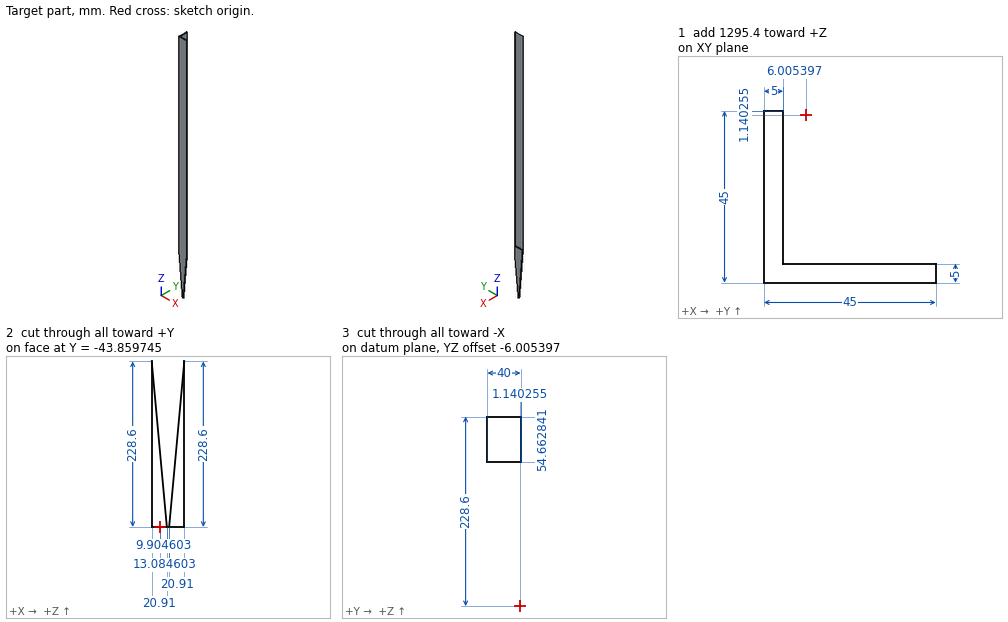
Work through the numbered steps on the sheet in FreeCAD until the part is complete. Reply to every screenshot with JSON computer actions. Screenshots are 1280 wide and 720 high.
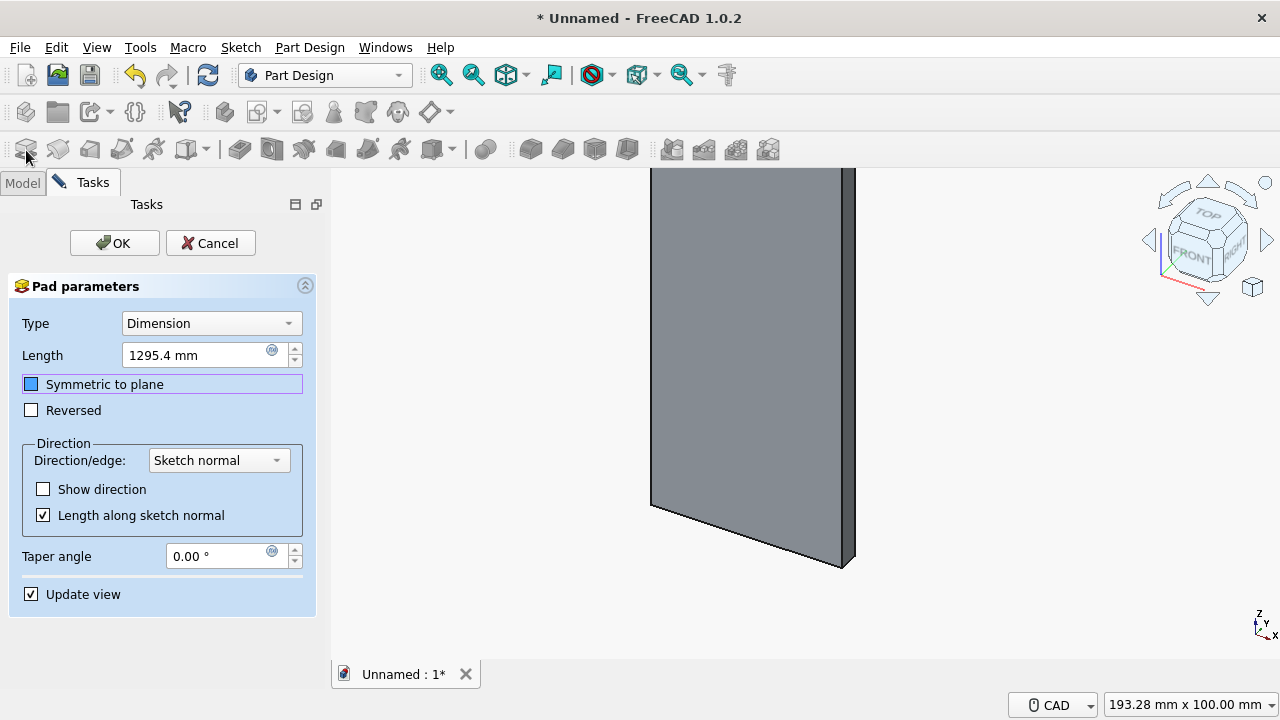
{"action": "left_click", "coordinate": [115, 243]}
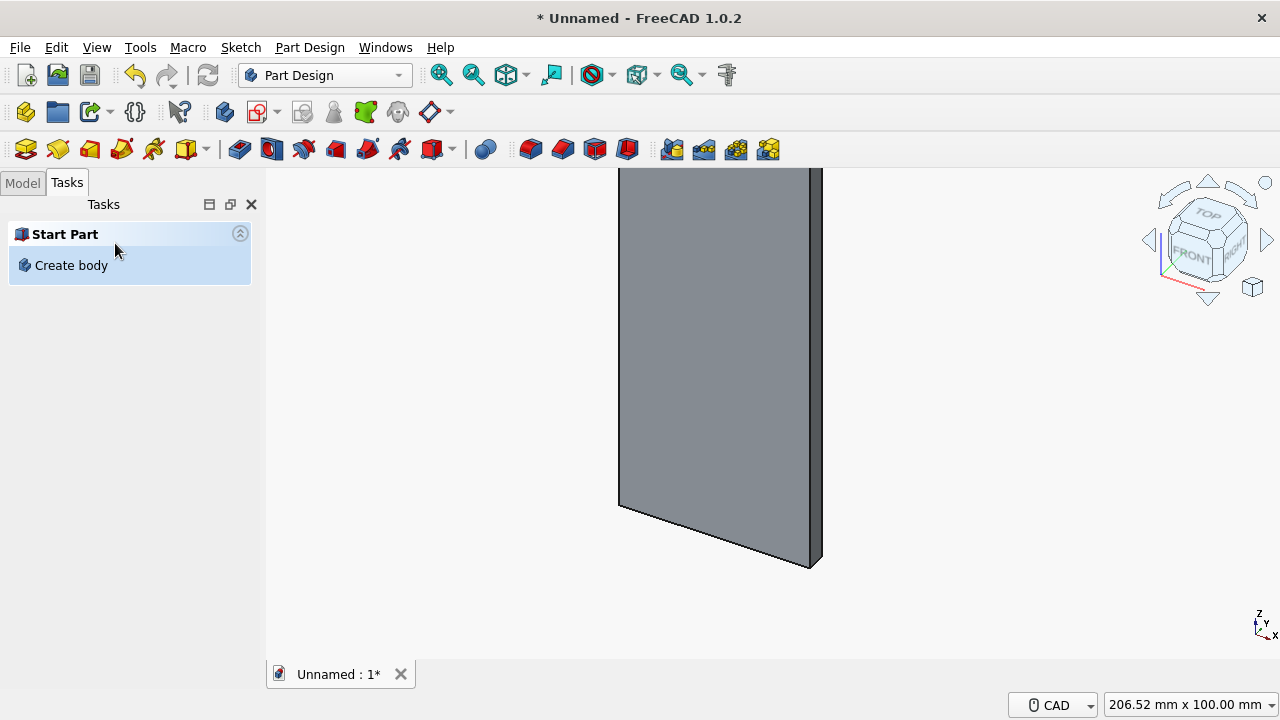
{"action": "left_click", "coordinate": [442, 76]}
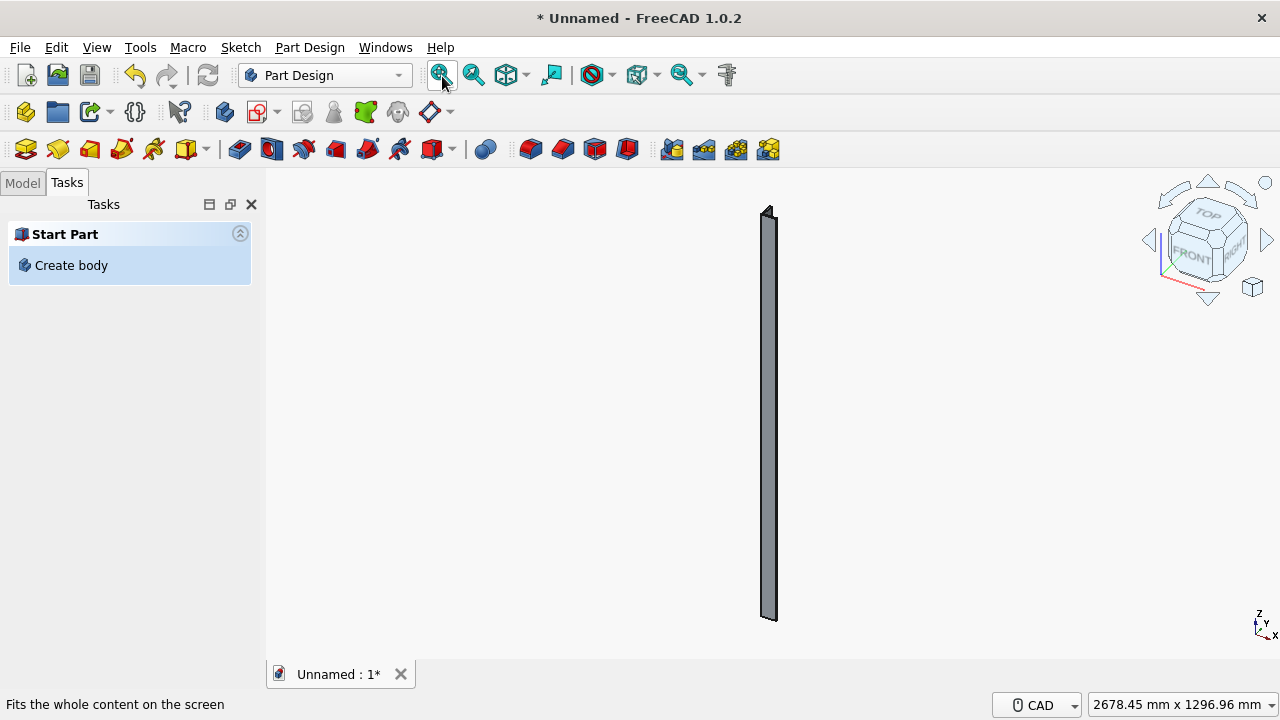
{"action": "left_click", "coordinate": [767, 244]}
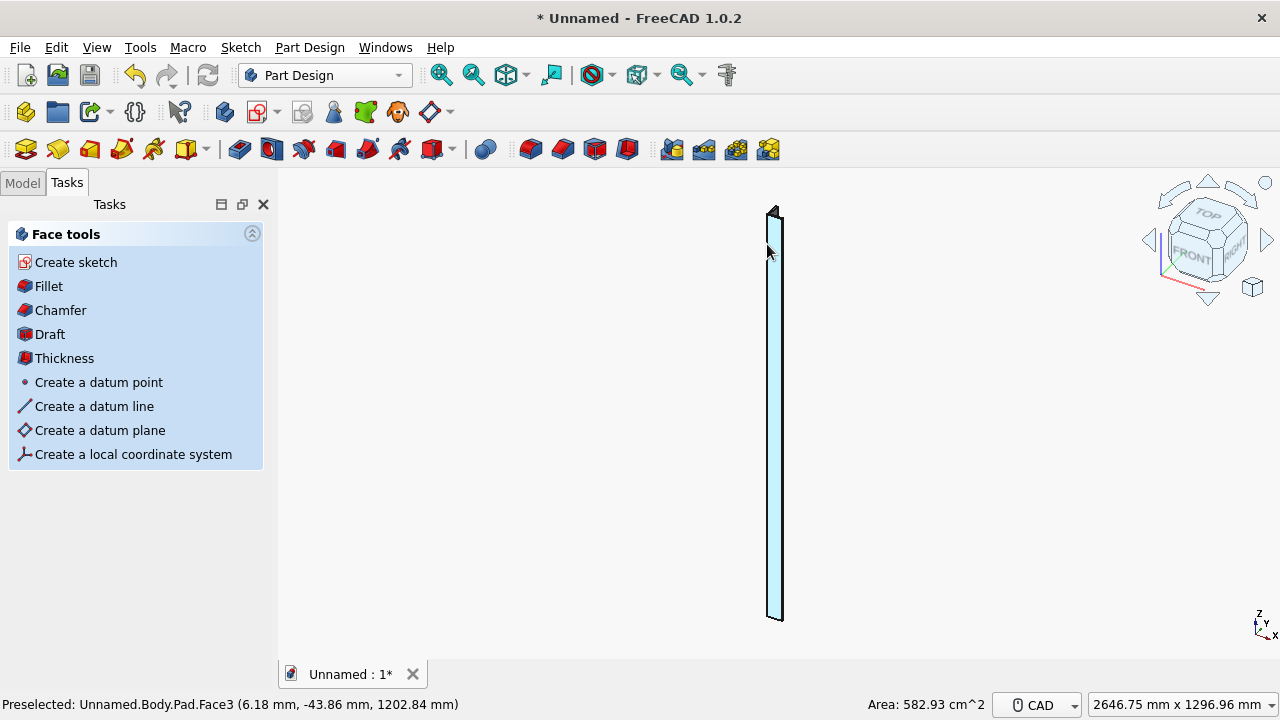
{"action": "left_click", "coordinate": [258, 112]}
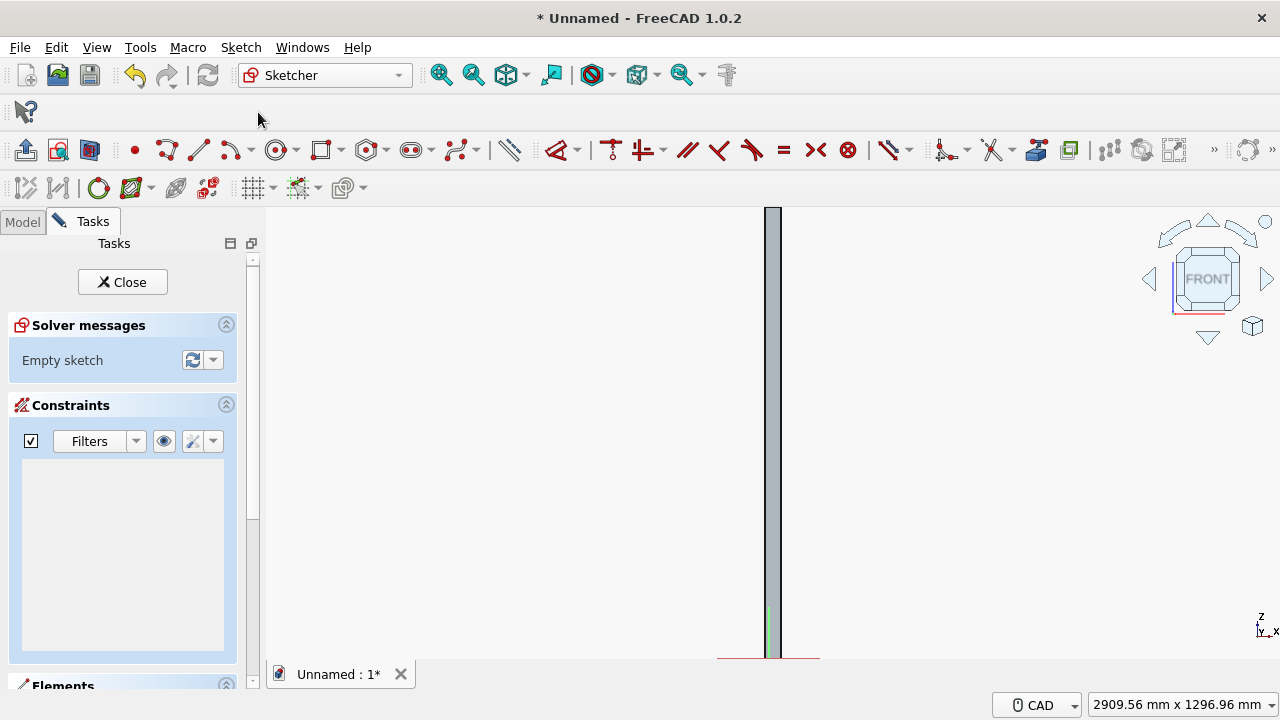
{"action": "scroll", "coordinate": [704, 433], "scroll_direction": "down", "scroll_amount": 5}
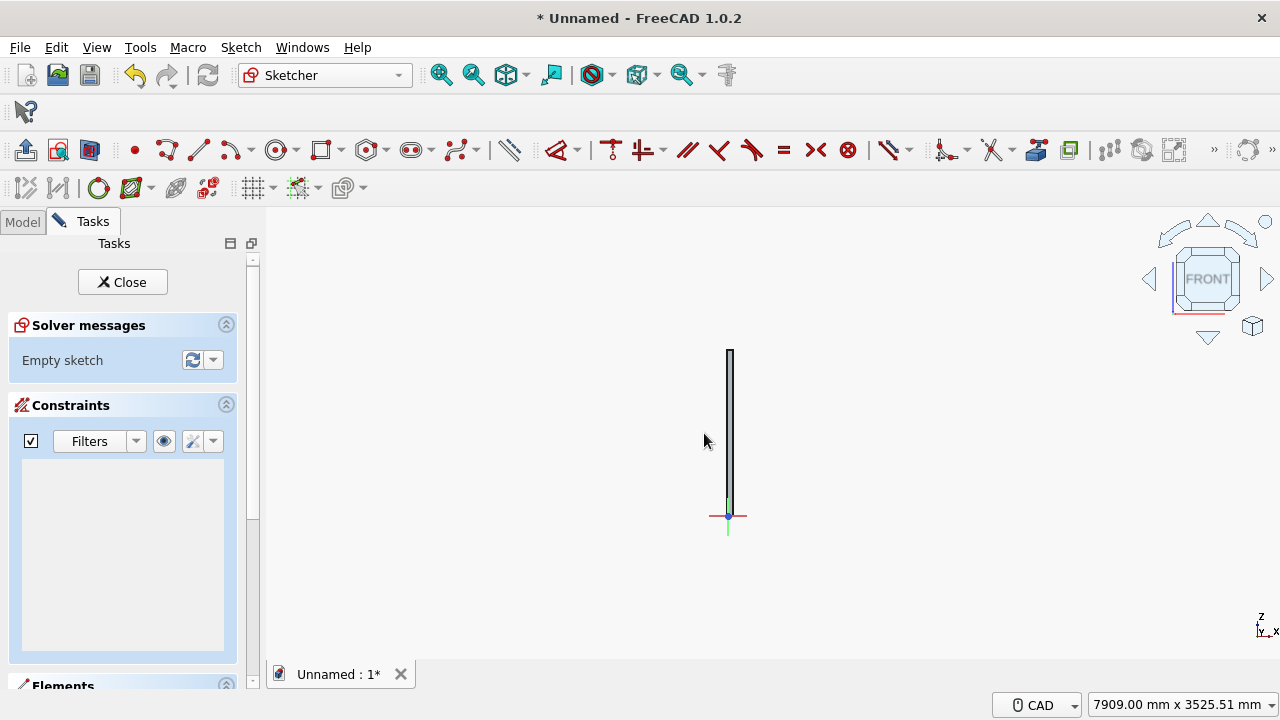
{"action": "scroll", "coordinate": [733, 510], "scroll_direction": "up", "scroll_amount": 11}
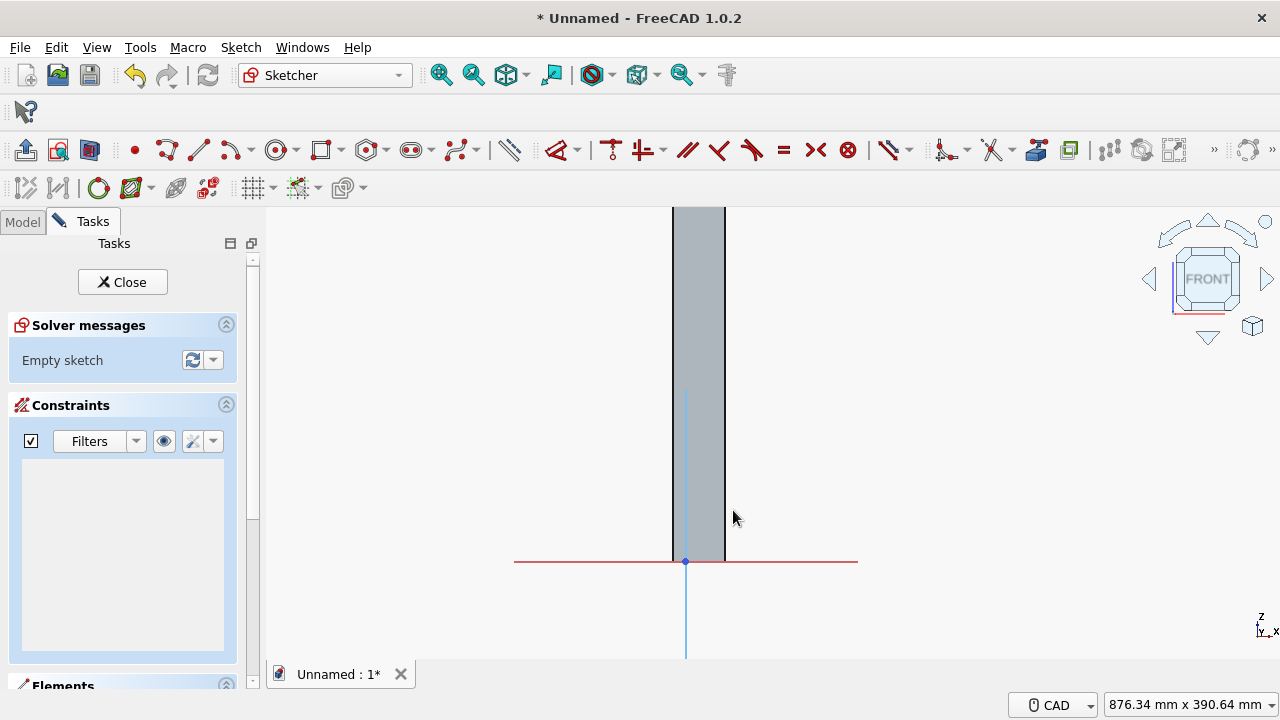
{"action": "left_click", "coordinate": [168, 150]}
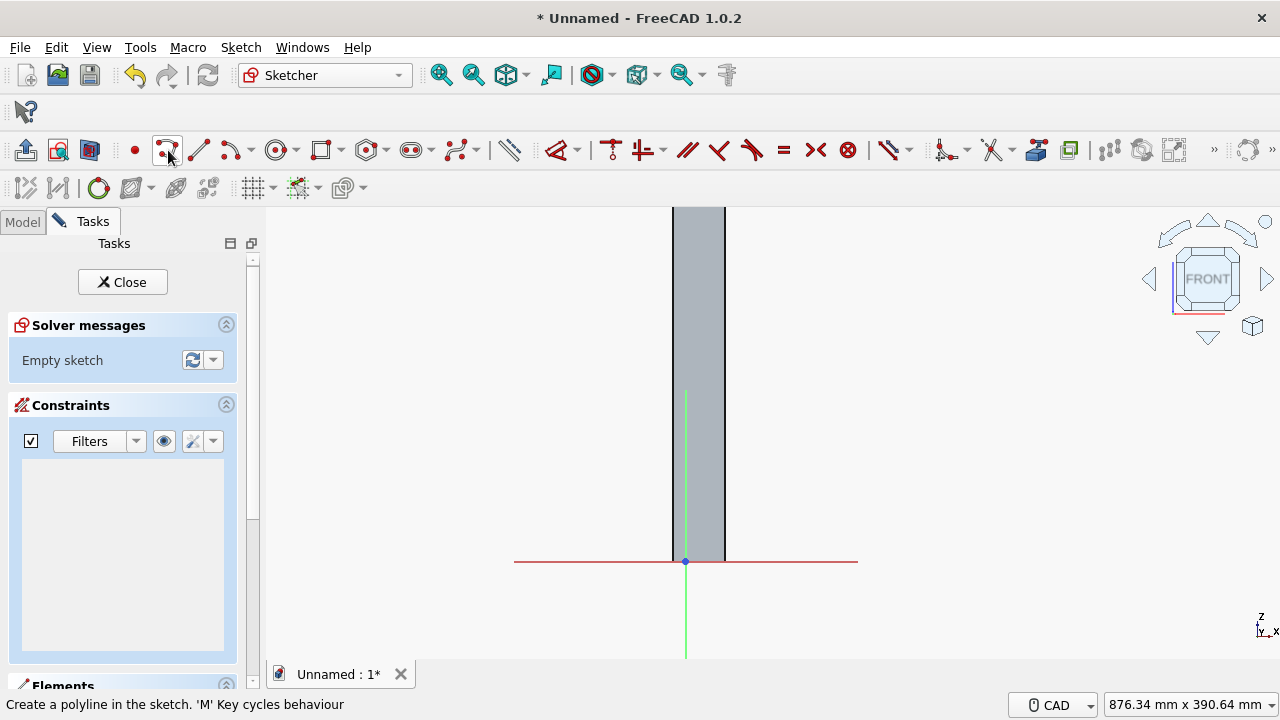
{"action": "scroll", "coordinate": [697, 562], "scroll_direction": "up", "scroll_amount": 2}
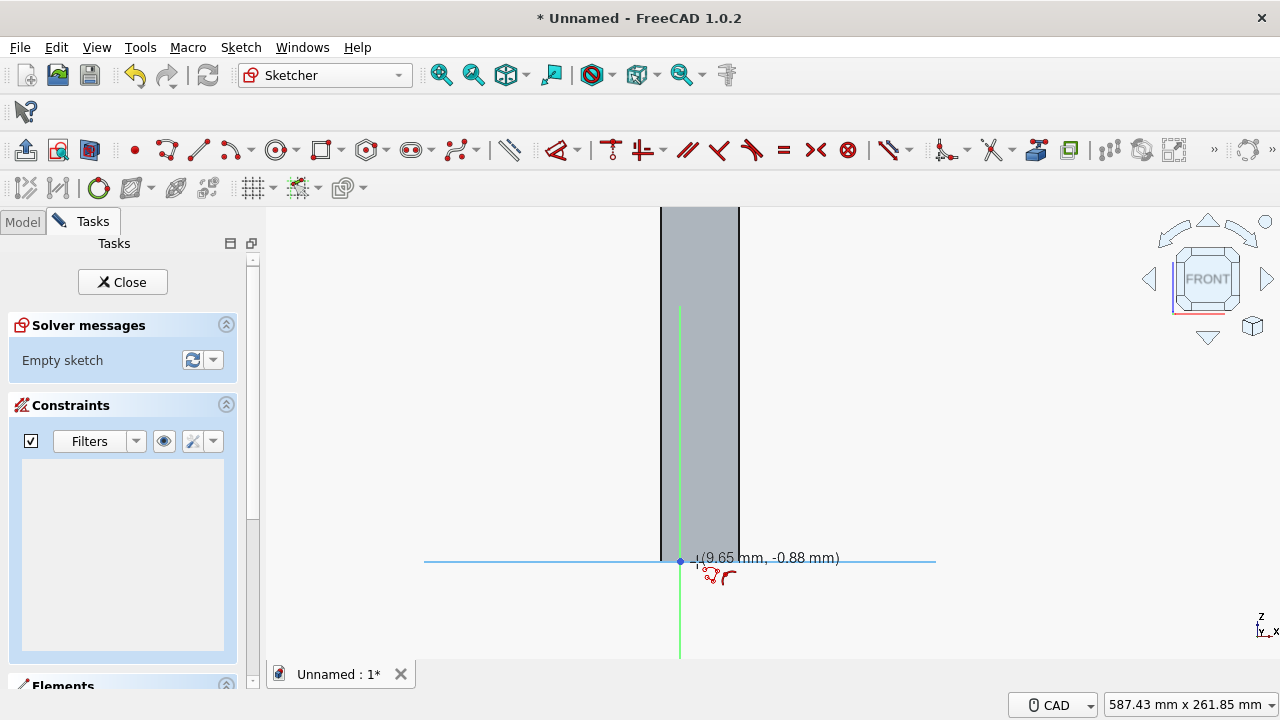
{"action": "left_click", "coordinate": [697, 562]}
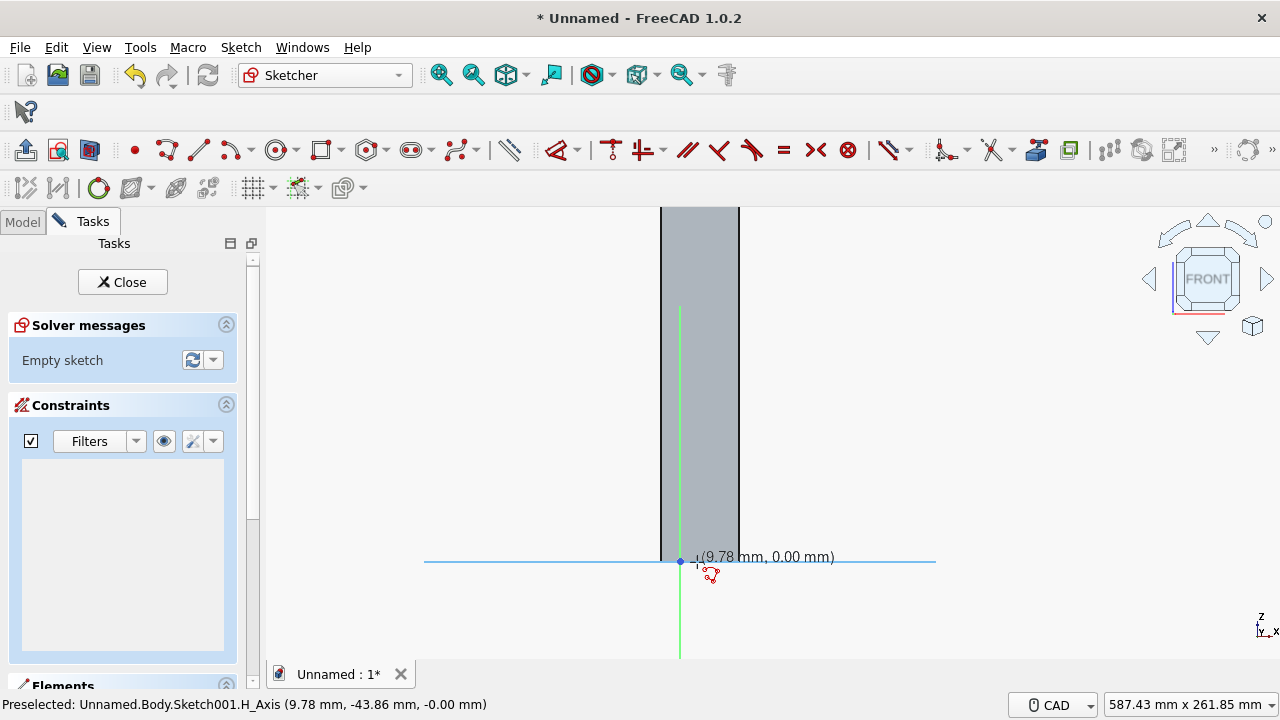
{"action": "scroll", "coordinate": [714, 573], "scroll_direction": "down", "scroll_amount": 2}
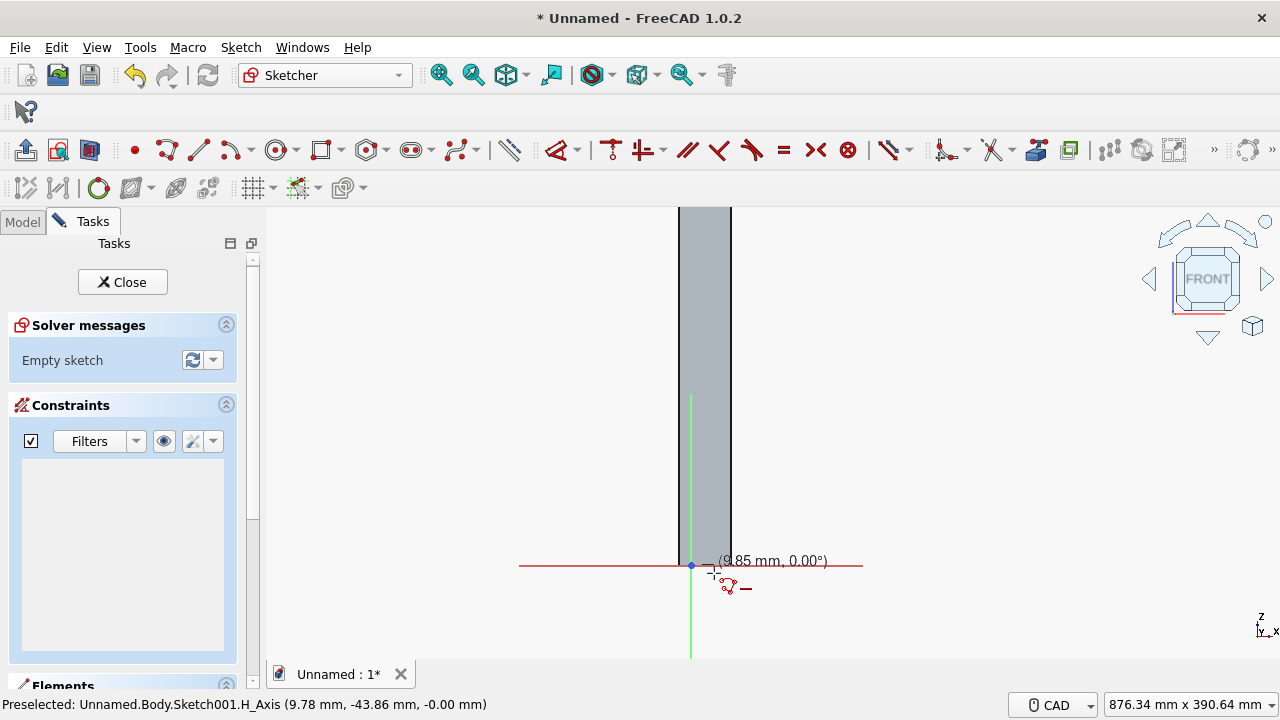
{"action": "scroll", "coordinate": [679, 301], "scroll_direction": "up", "scroll_amount": 2}